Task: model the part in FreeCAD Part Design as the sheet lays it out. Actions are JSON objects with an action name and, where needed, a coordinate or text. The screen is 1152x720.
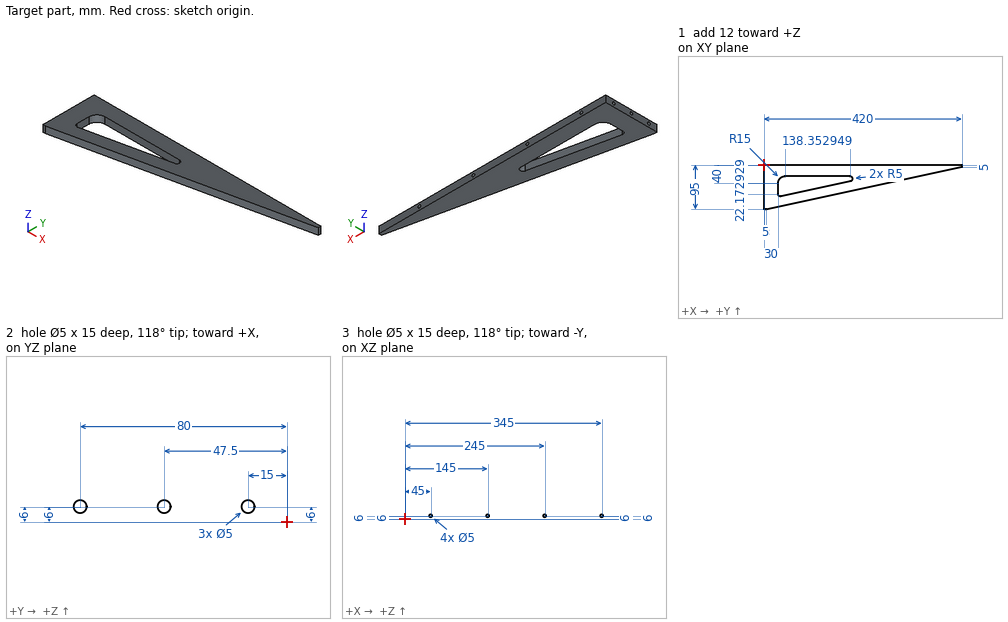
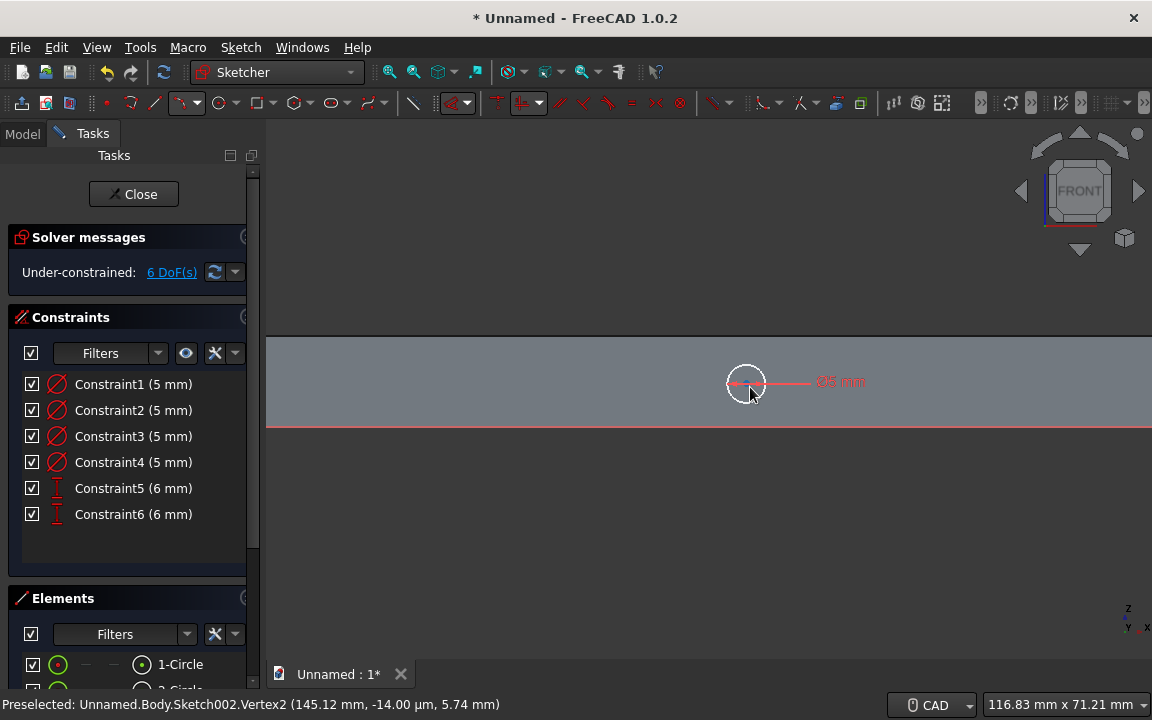
{"action": "left_click", "coordinate": [746, 384]}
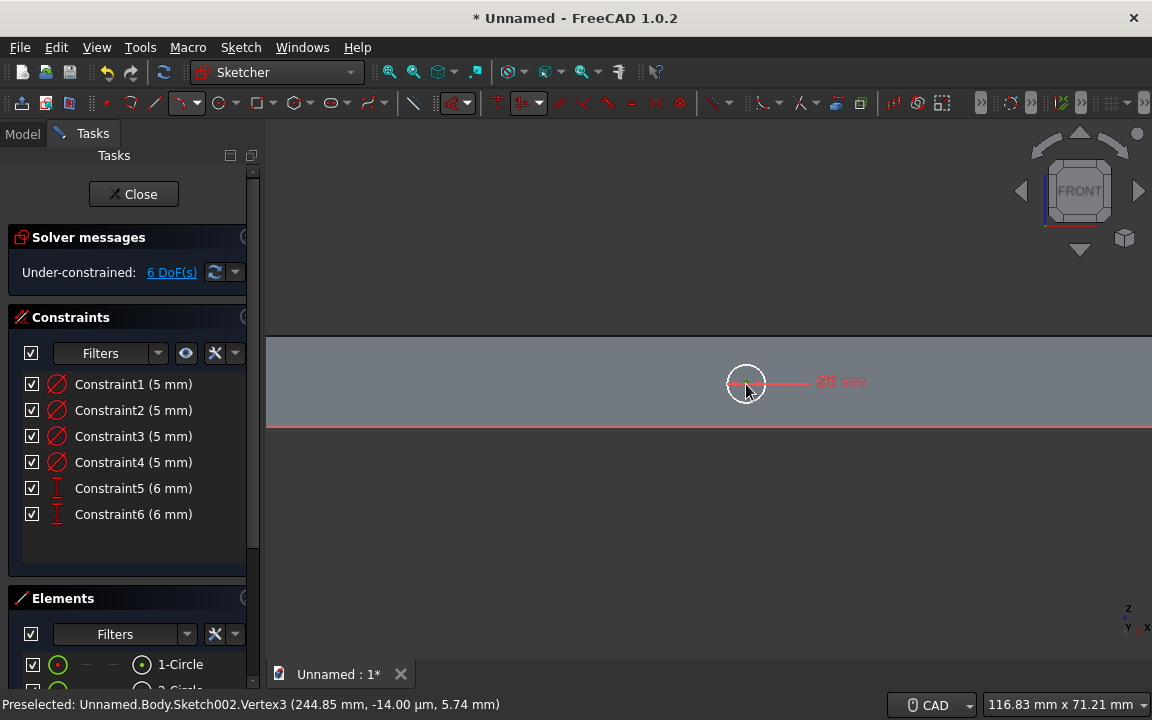
{"action": "key", "text": "i"}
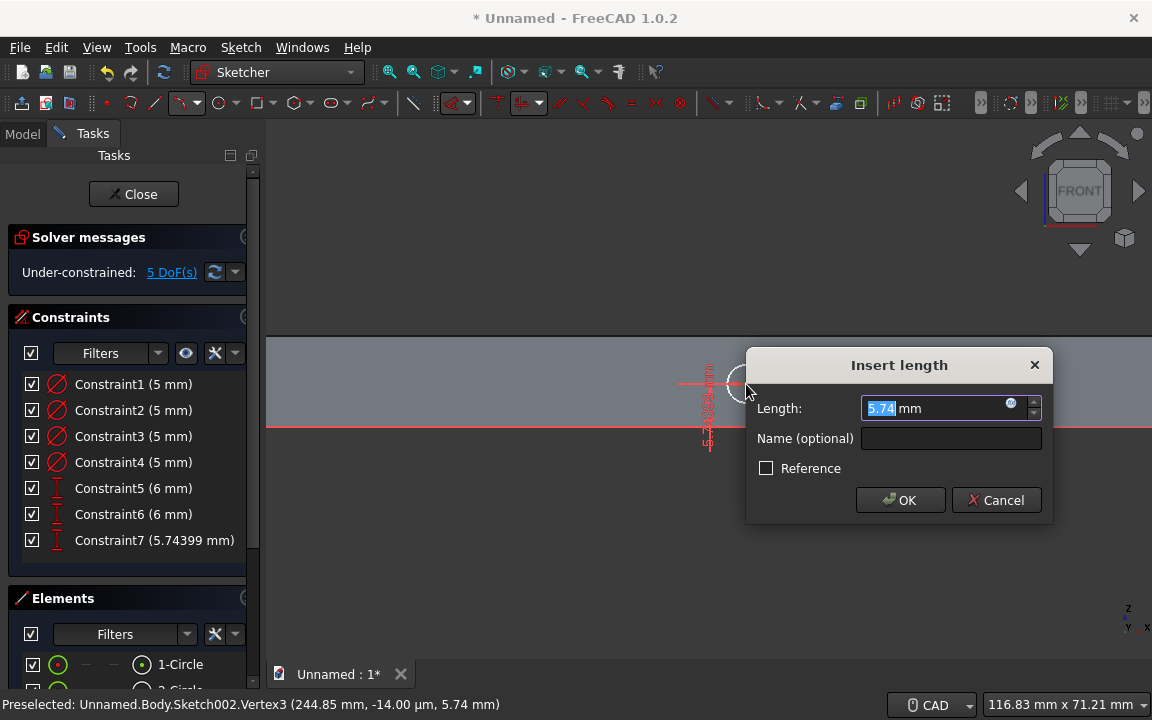
{"action": "type", "text": "6"}
{"action": "key", "text": "Return"}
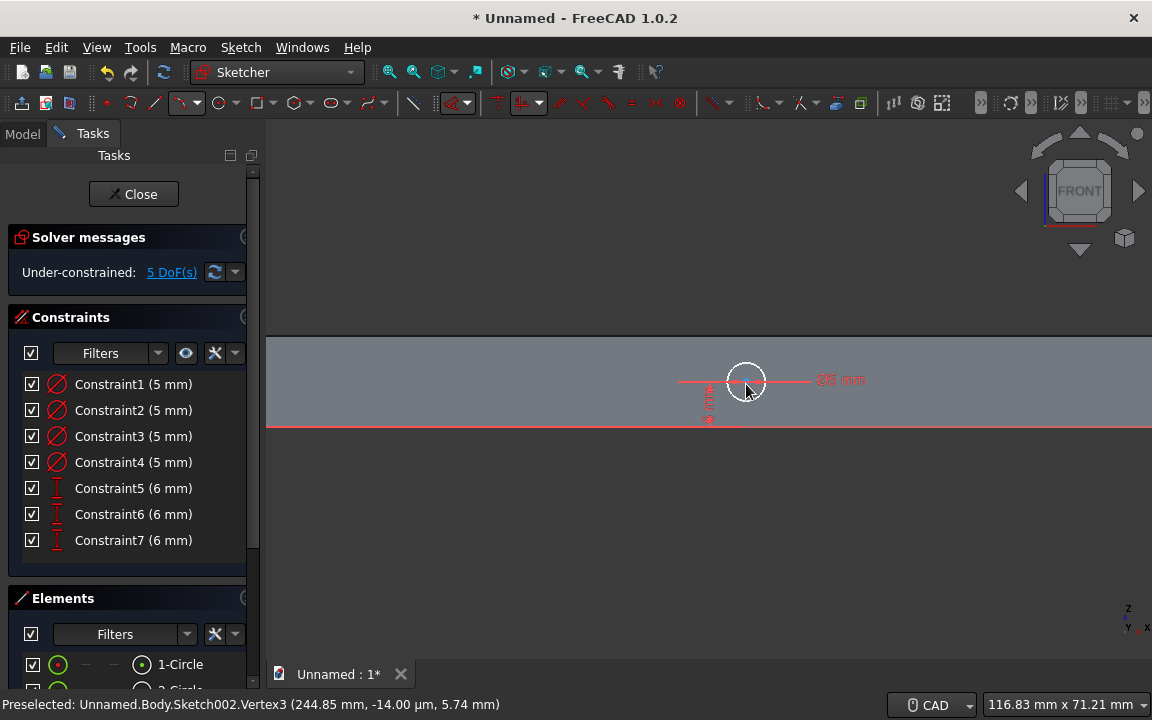
{"action": "scroll", "coordinate": [750, 387], "scroll_direction": "down", "scroll_amount": 8}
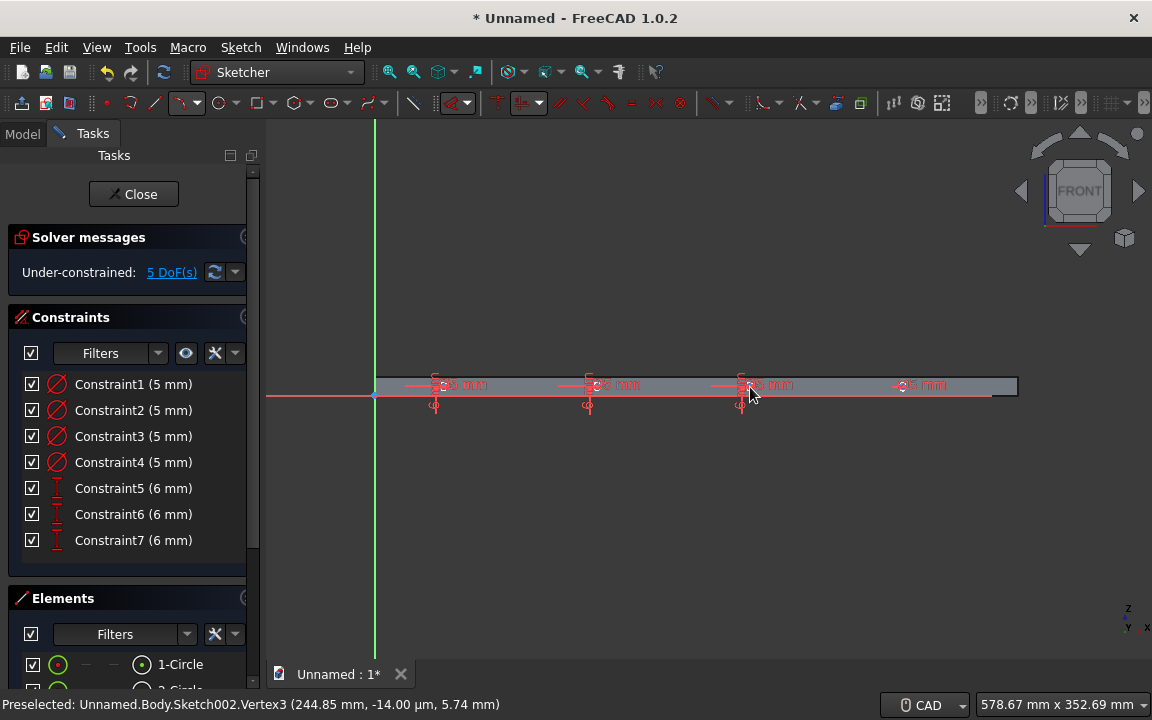
{"action": "scroll", "coordinate": [903, 387], "scroll_direction": "up", "scroll_amount": 8}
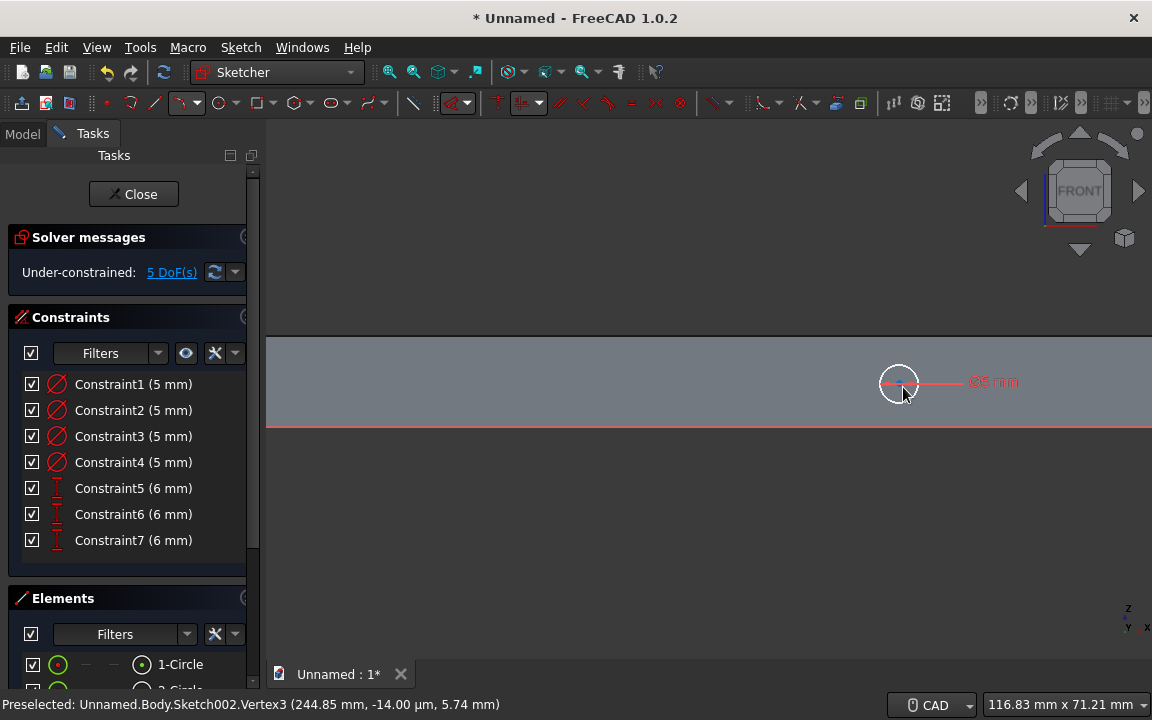
{"action": "left_click", "coordinate": [899, 384]}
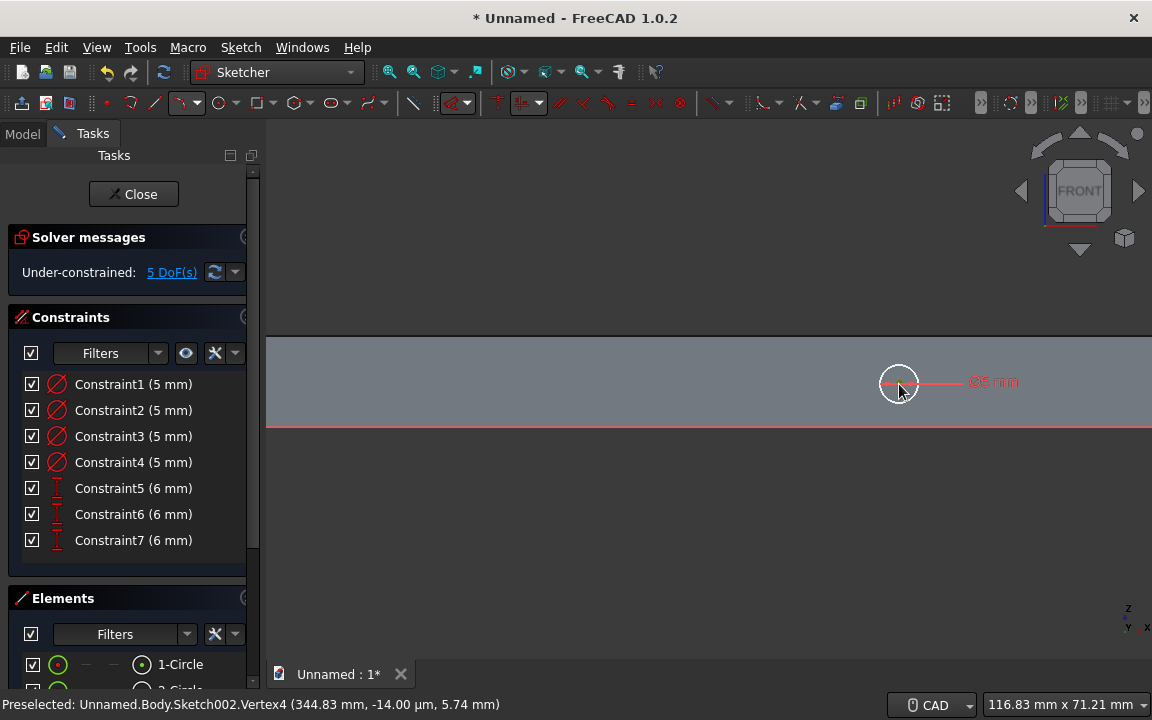
{"action": "key", "text": "i"}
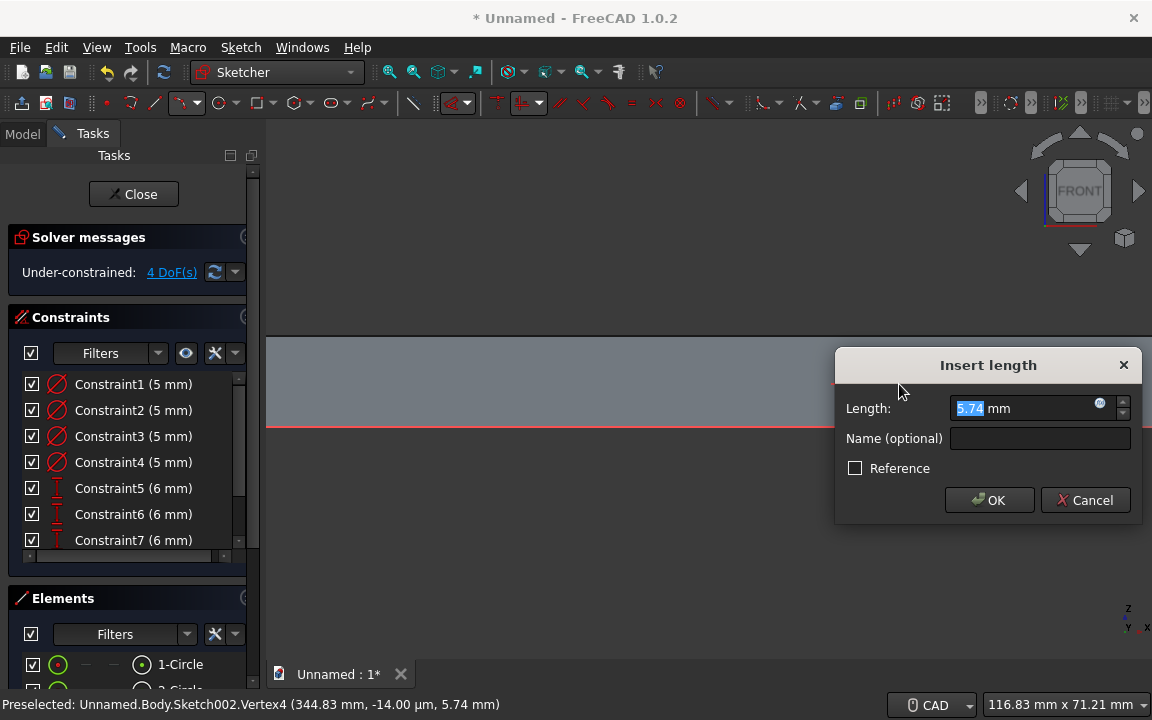
{"action": "type", "text": "6"}
{"action": "key", "text": "Return"}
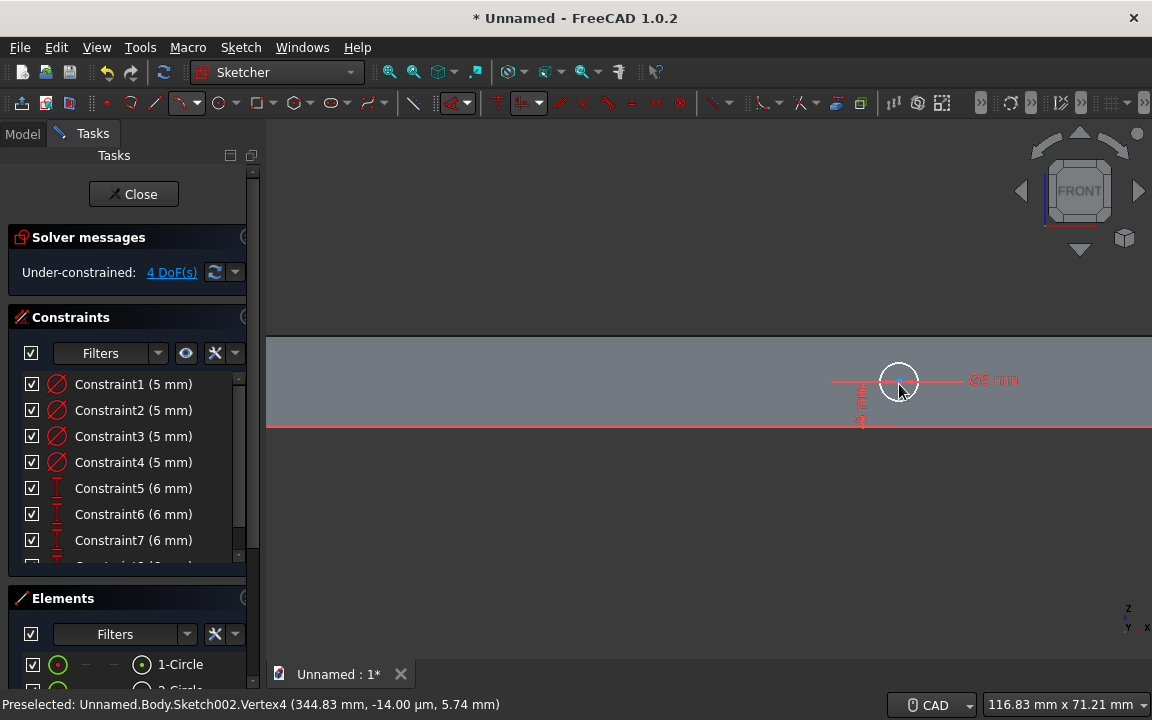
{"action": "scroll", "coordinate": [903, 387], "scroll_direction": "down", "scroll_amount": 8}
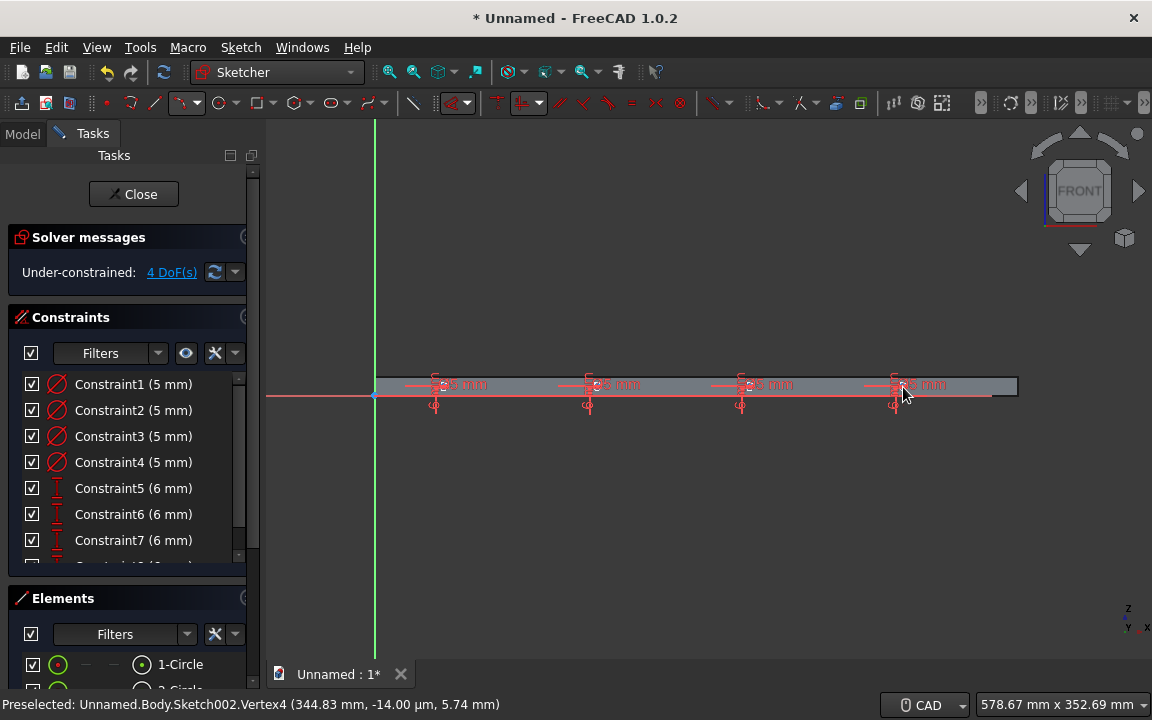
{"action": "left_click", "coordinate": [444, 386]}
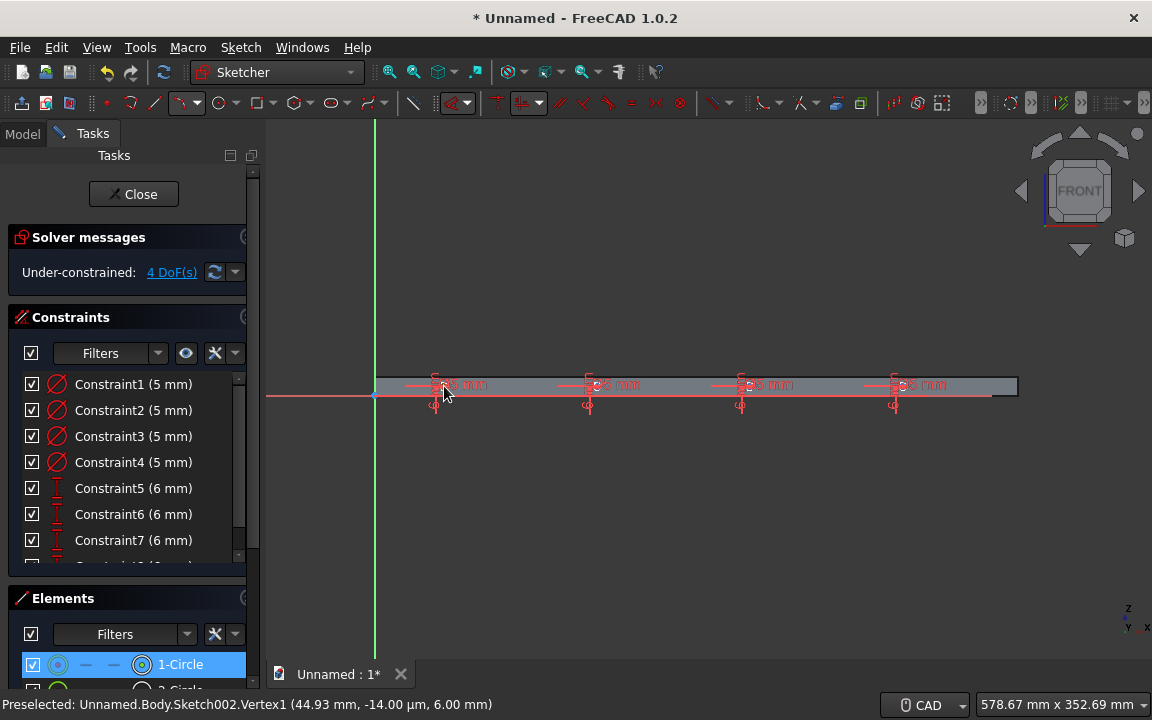
{"action": "left_click", "coordinate": [470, 104]}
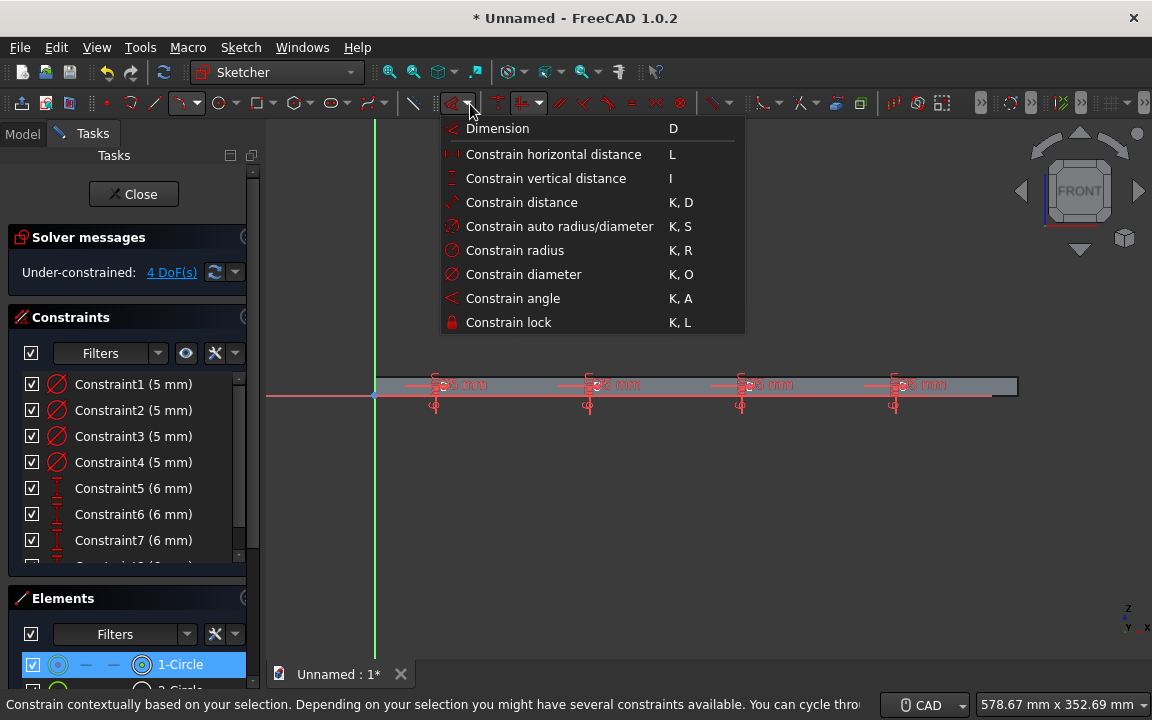
{"action": "left_click", "coordinate": [593, 154]}